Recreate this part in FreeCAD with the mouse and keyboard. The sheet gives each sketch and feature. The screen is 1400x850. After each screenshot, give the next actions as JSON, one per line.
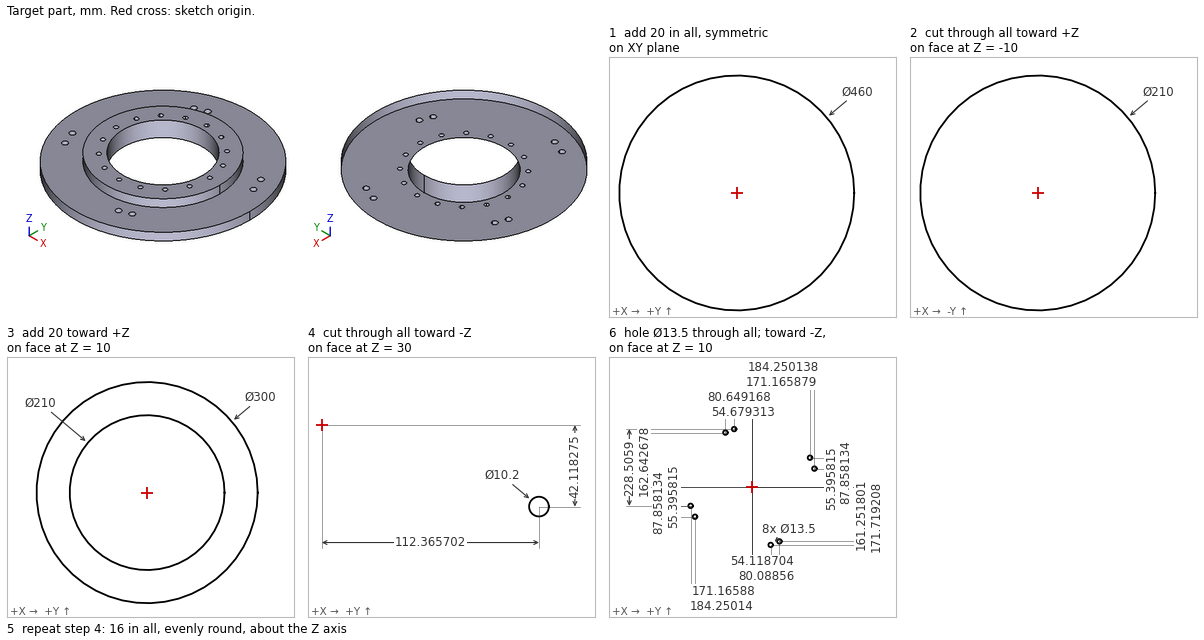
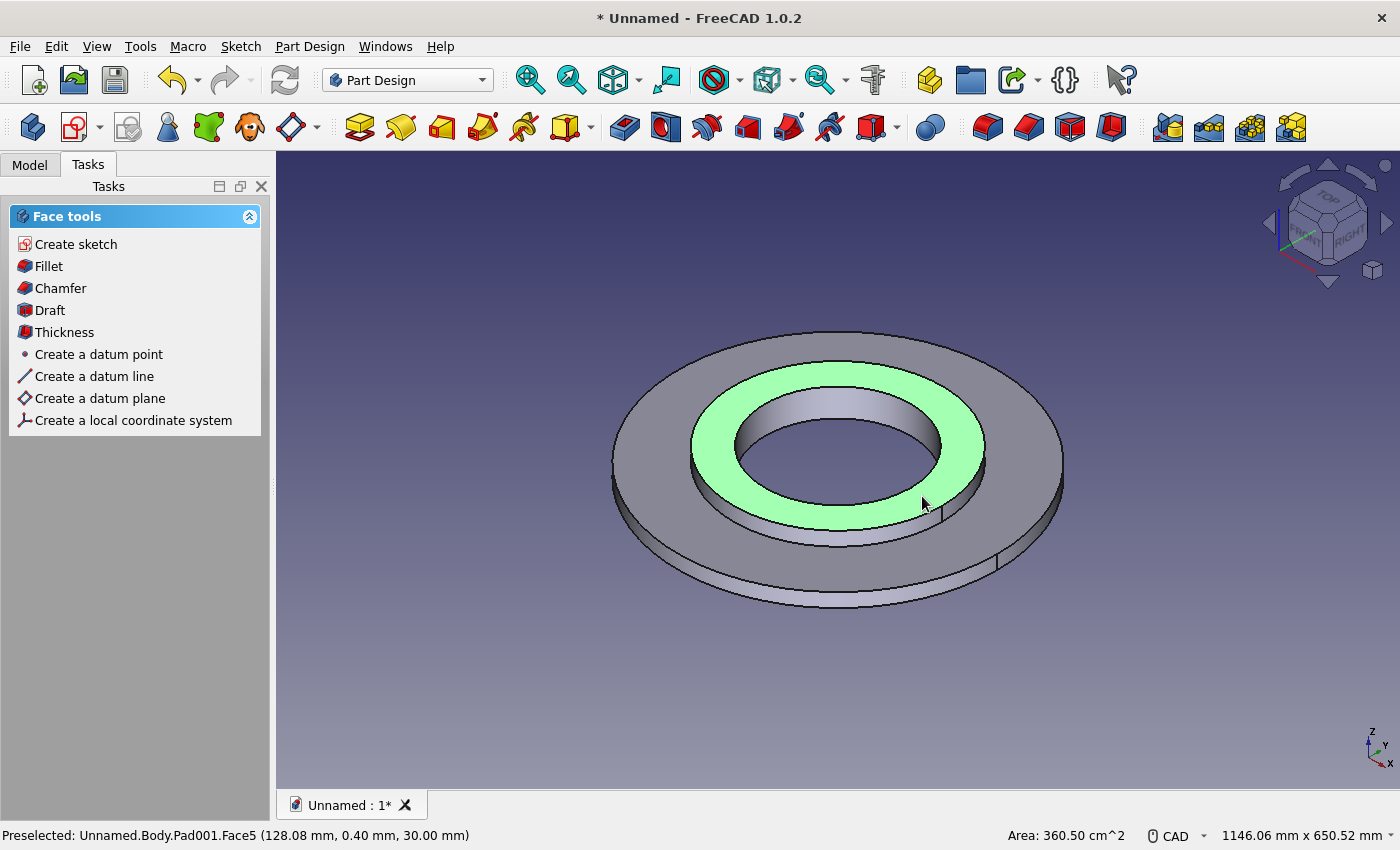
{"action": "left_click", "coordinate": [74, 128]}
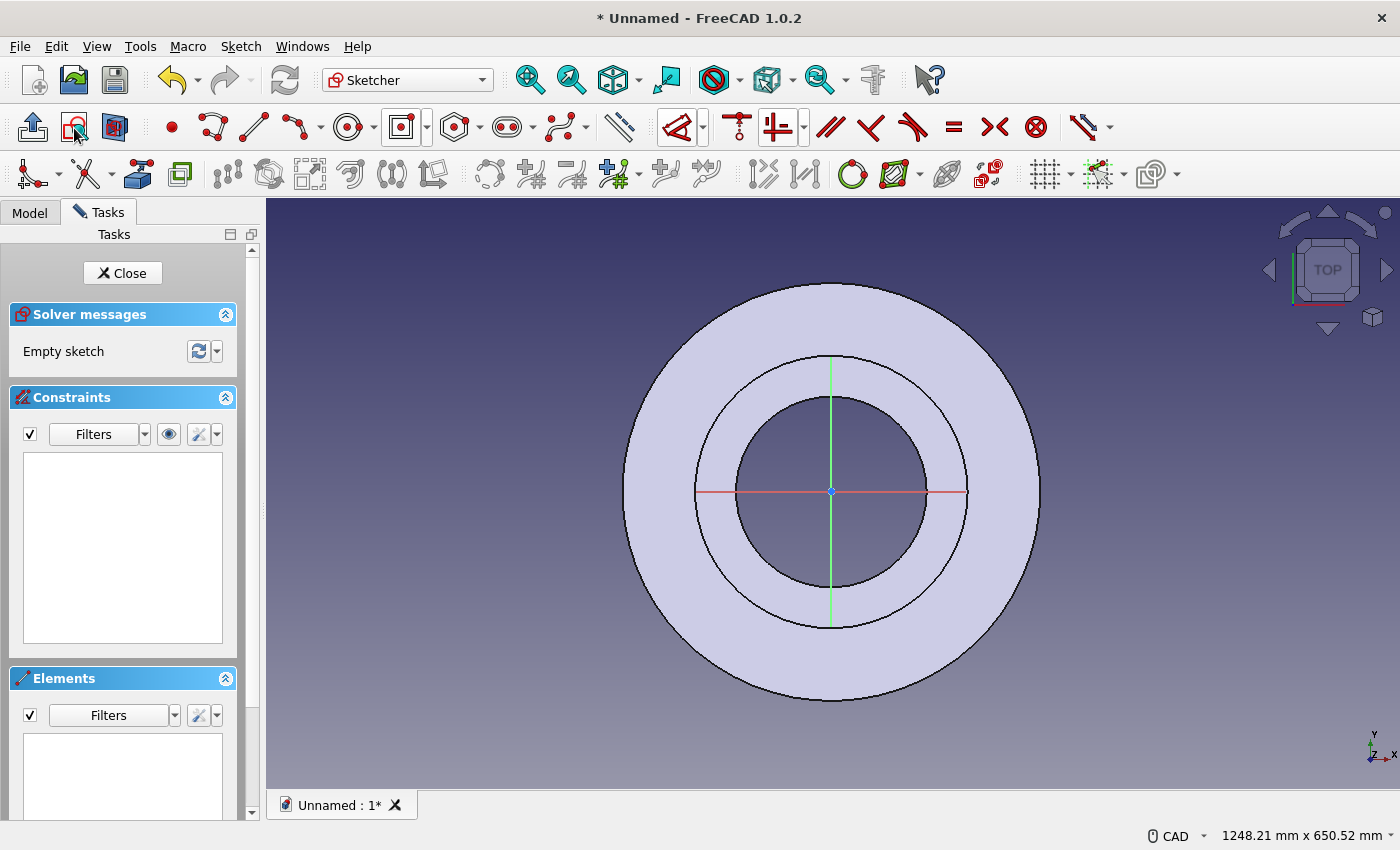
{"action": "scroll", "coordinate": [942, 532], "scroll_direction": "up", "scroll_amount": 15}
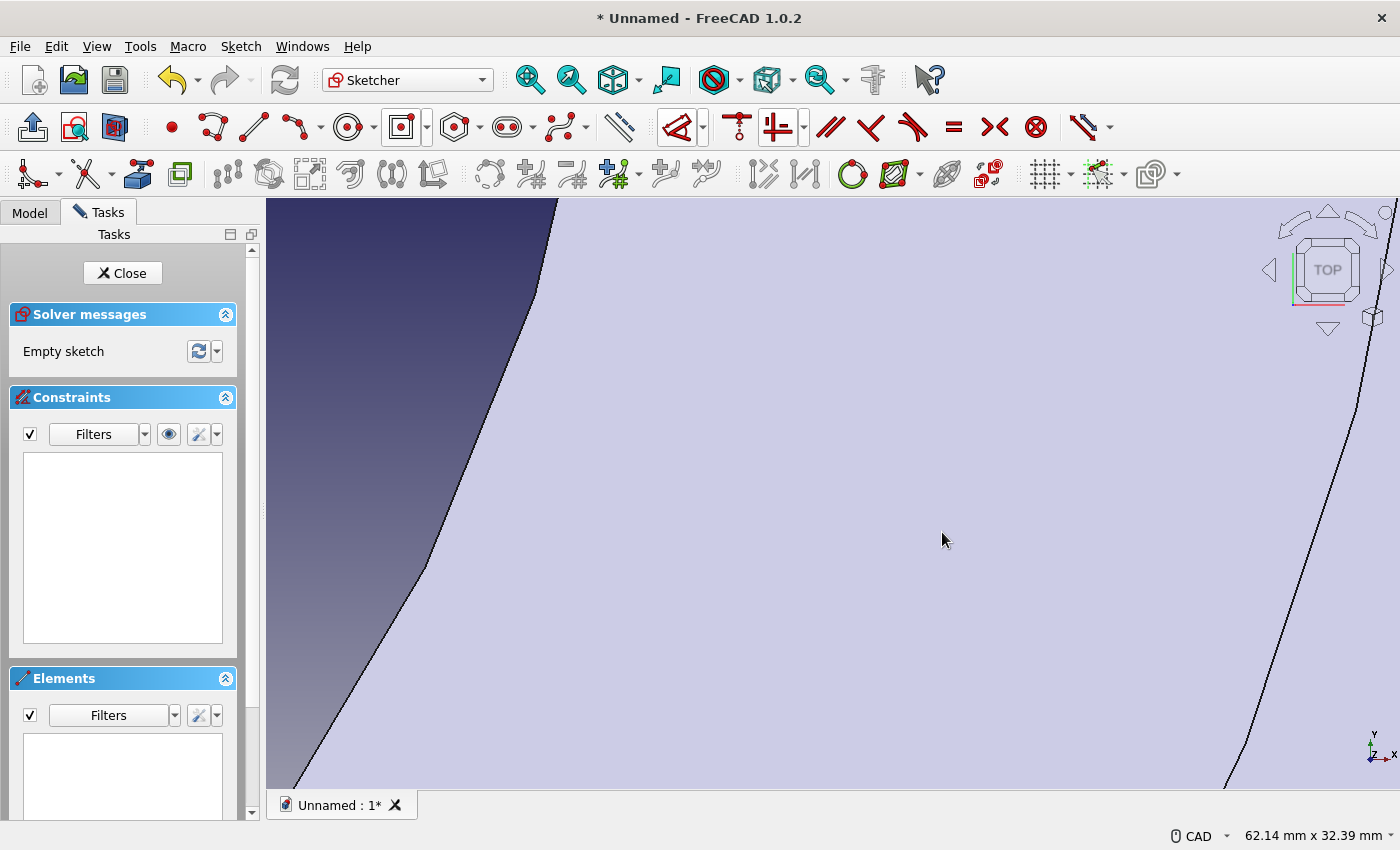
{"action": "scroll", "coordinate": [754, 480], "scroll_direction": "up", "scroll_amount": 4}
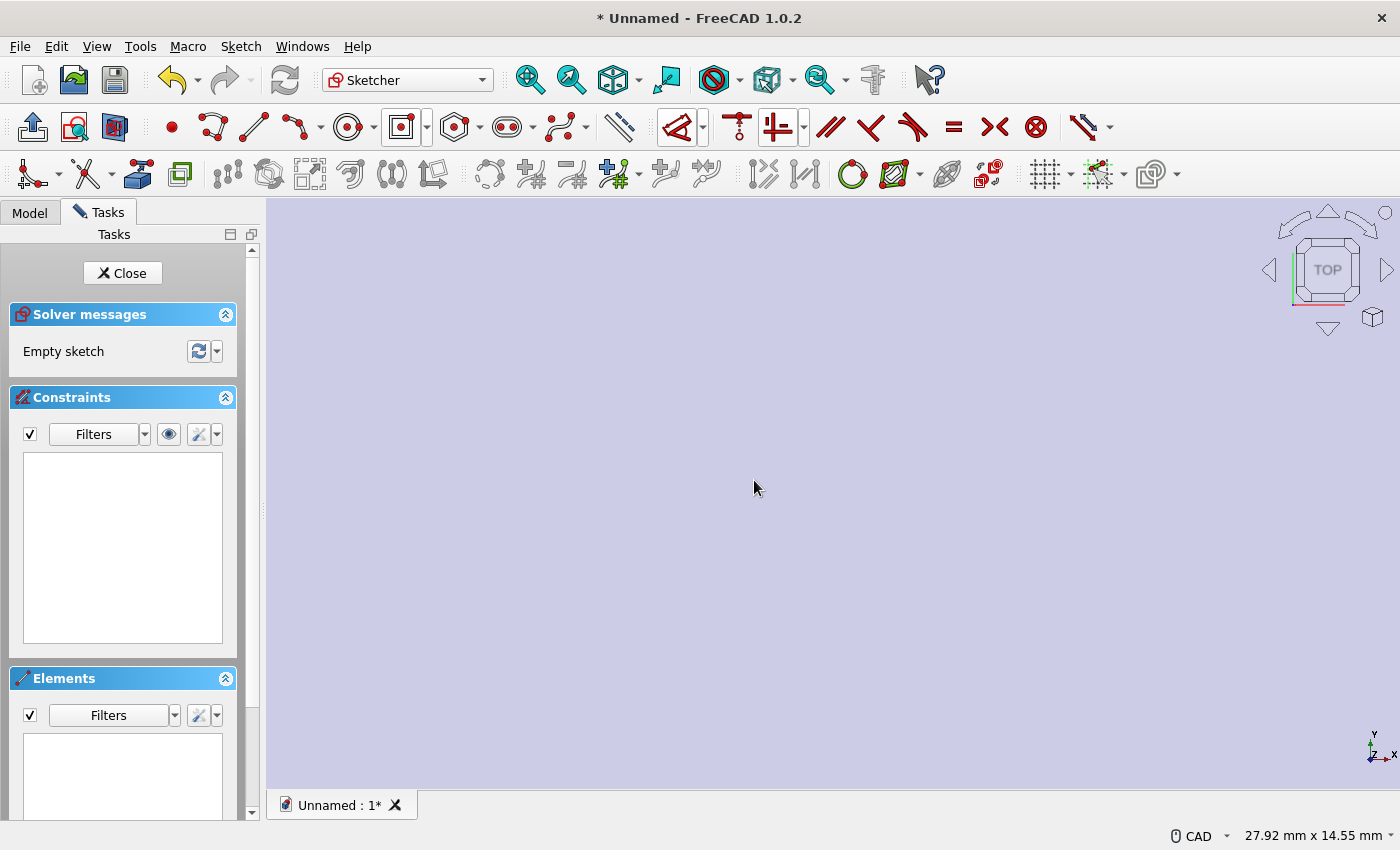
{"action": "key", "text": "g c"}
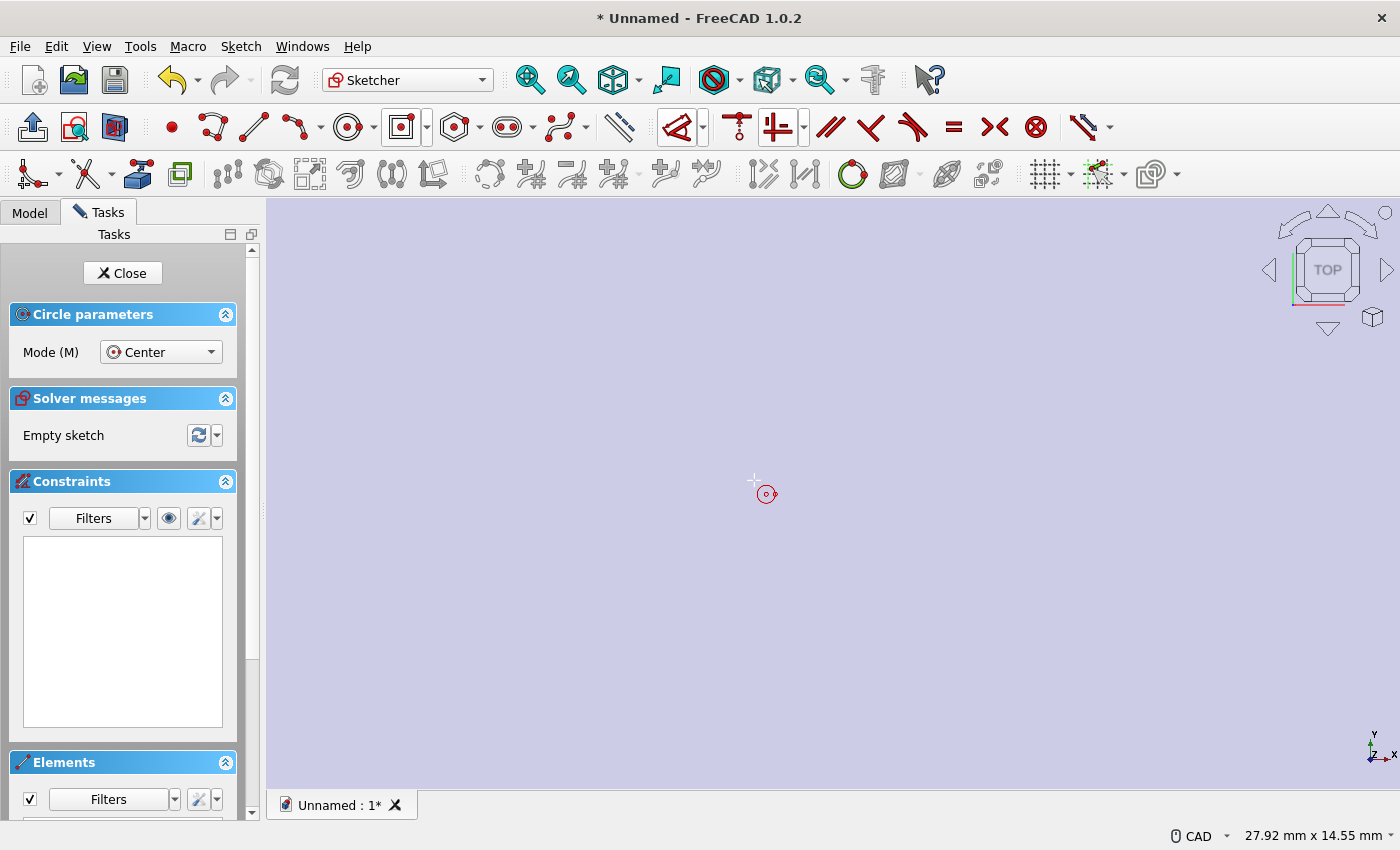
{"action": "left_click", "coordinate": [763, 493]}
{"action": "mouse_move", "coordinate": [910, 346]}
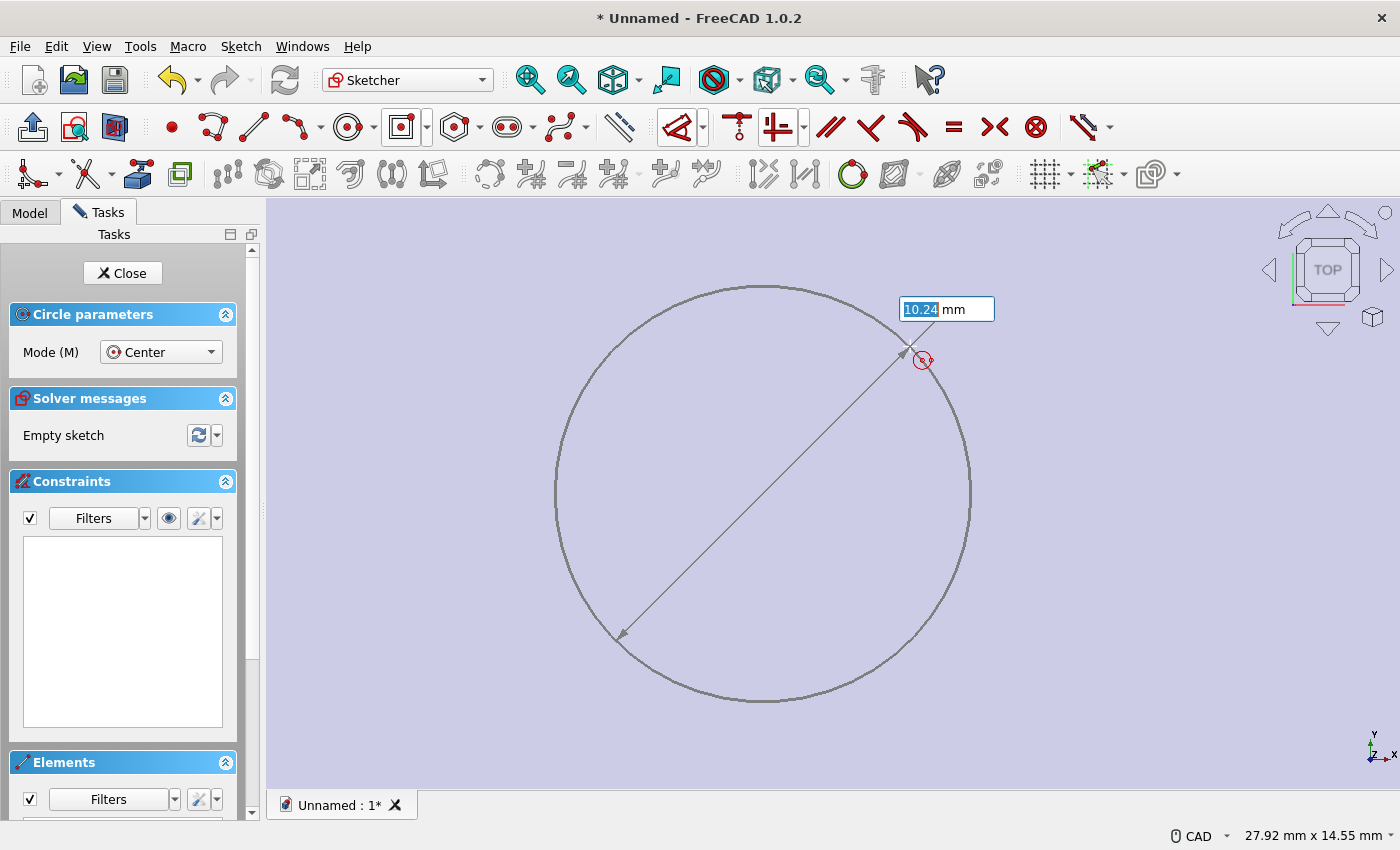
{"action": "type", "text": "10.2"}
{"action": "key", "text": "Return"}
{"action": "key", "text": "Escape"}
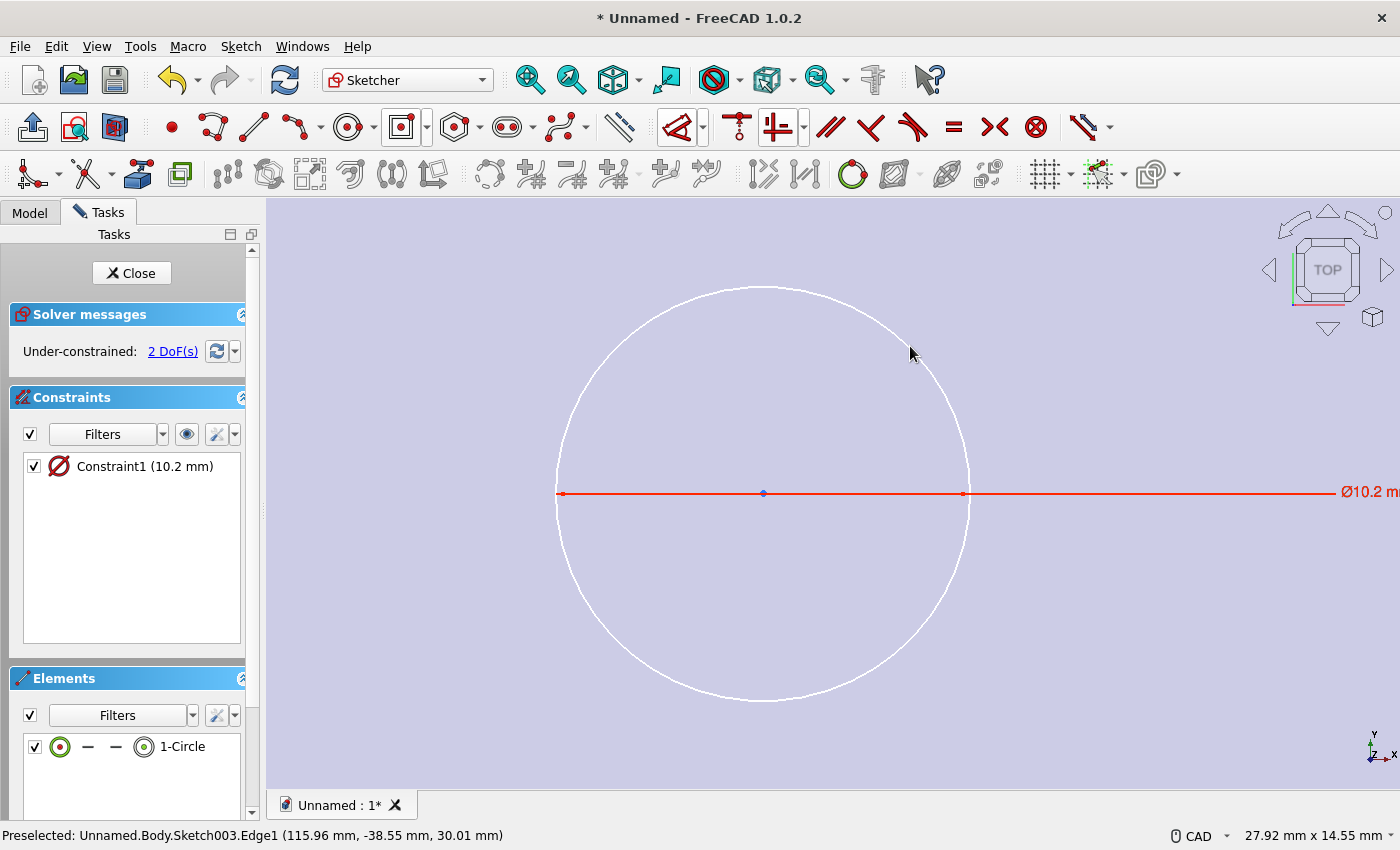
{"action": "left_click", "coordinate": [676, 128]}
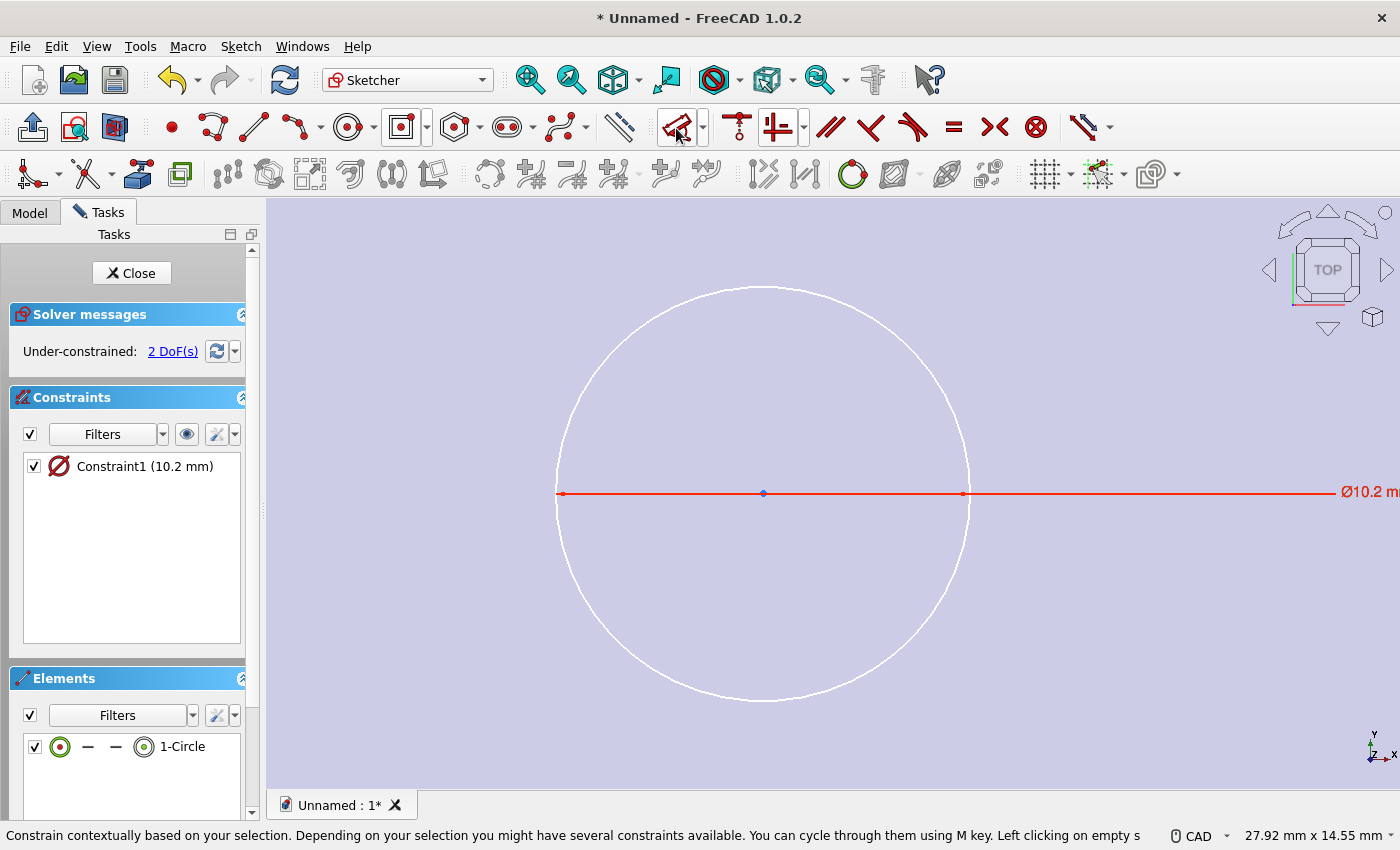
{"action": "left_click", "coordinate": [763, 494]}
{"action": "left_click", "coordinate": [797, 360]}